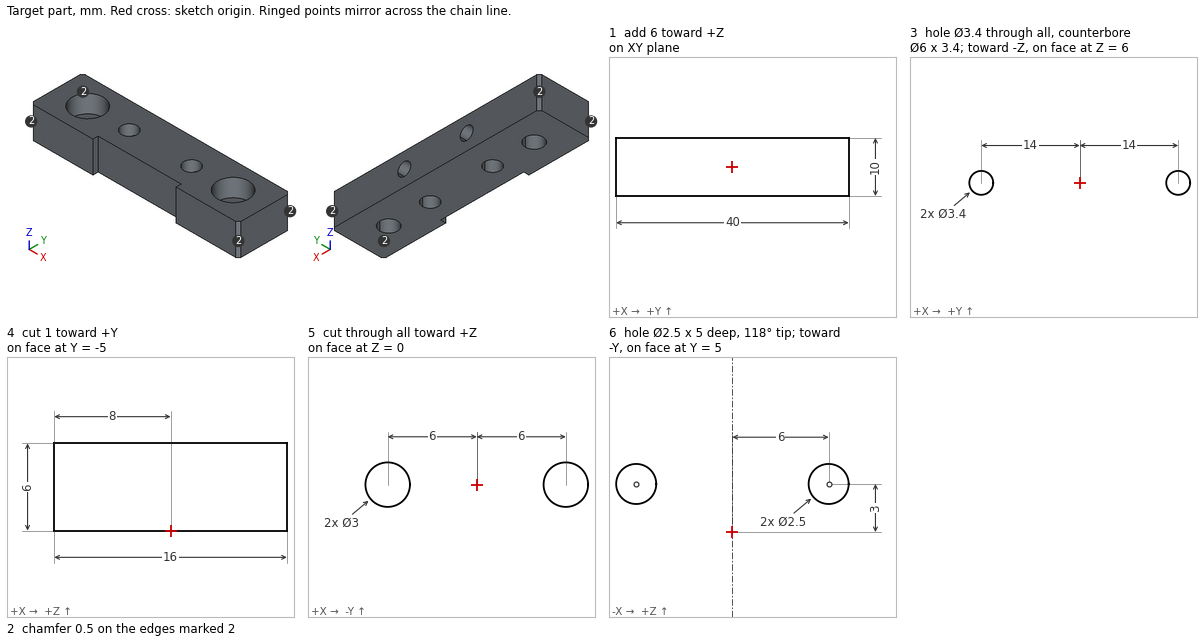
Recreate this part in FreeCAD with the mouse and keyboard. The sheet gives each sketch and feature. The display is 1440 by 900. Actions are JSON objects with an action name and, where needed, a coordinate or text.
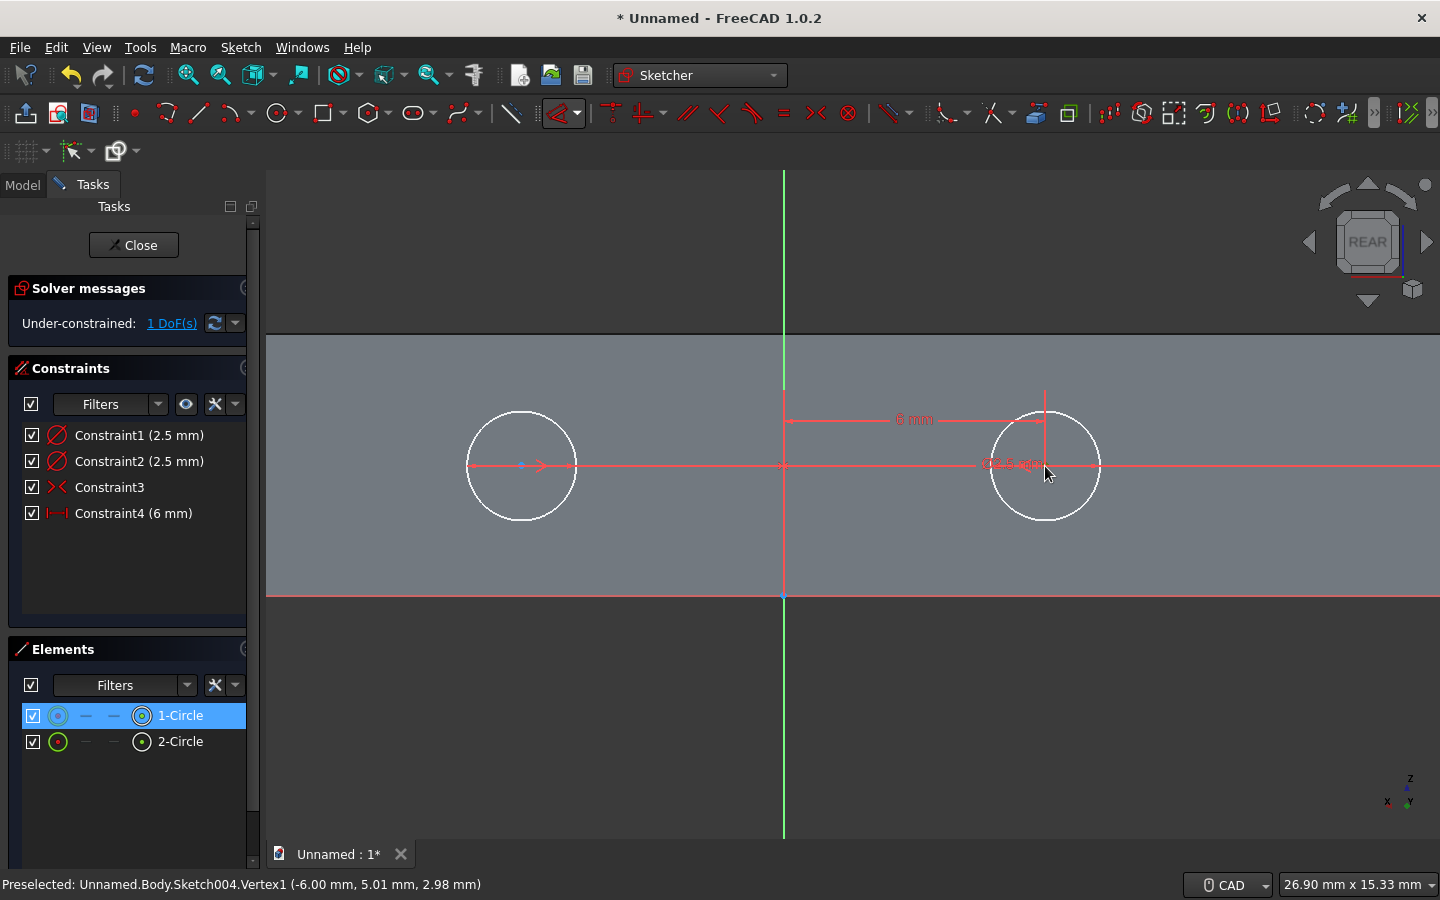
{"action": "left_click", "coordinate": [580, 114]}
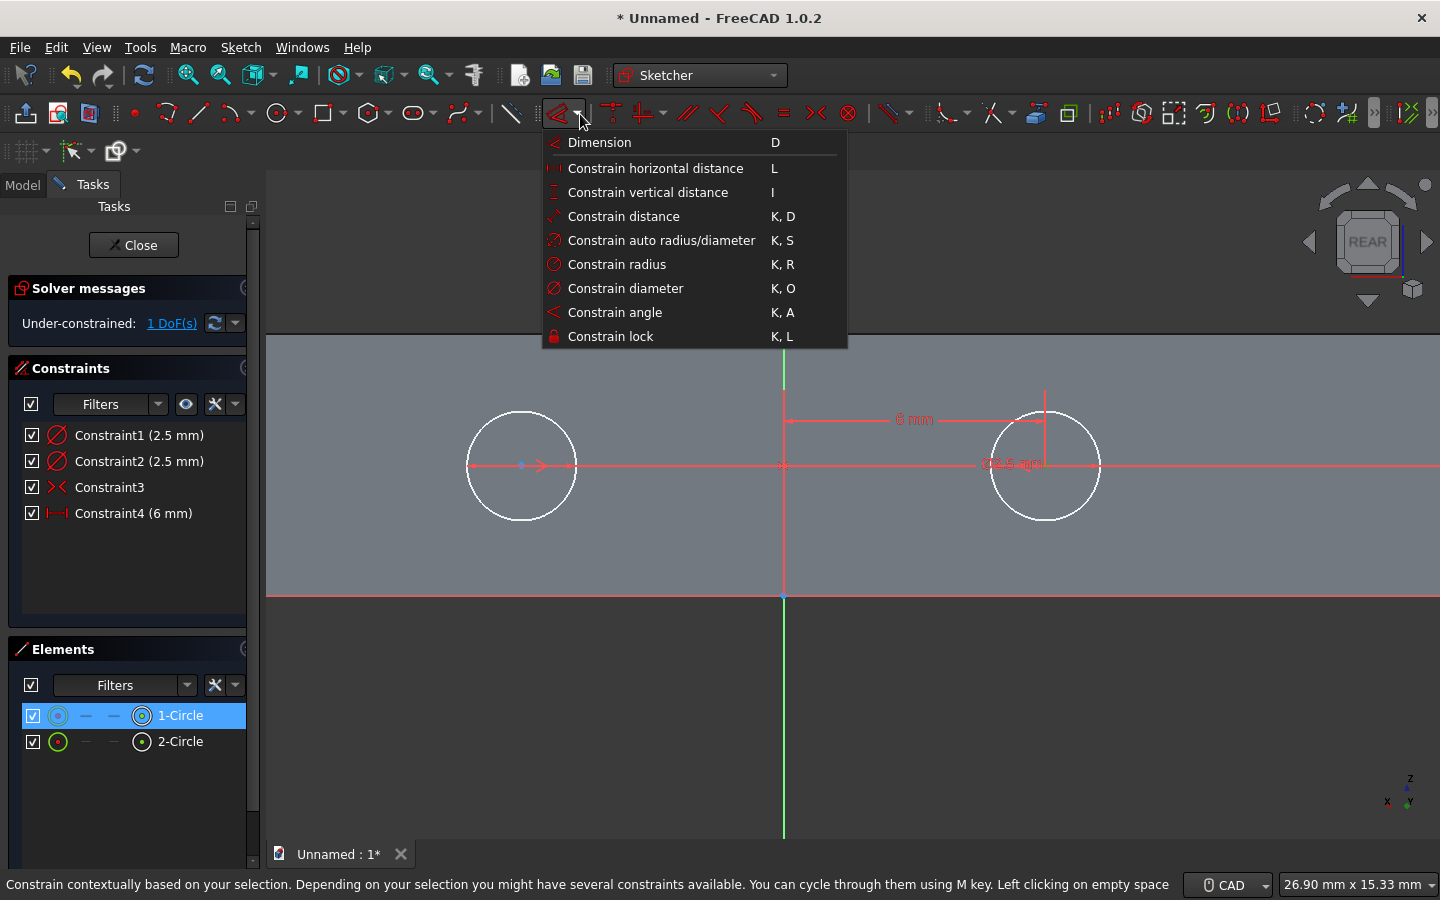
{"action": "left_click", "coordinate": [695, 192]}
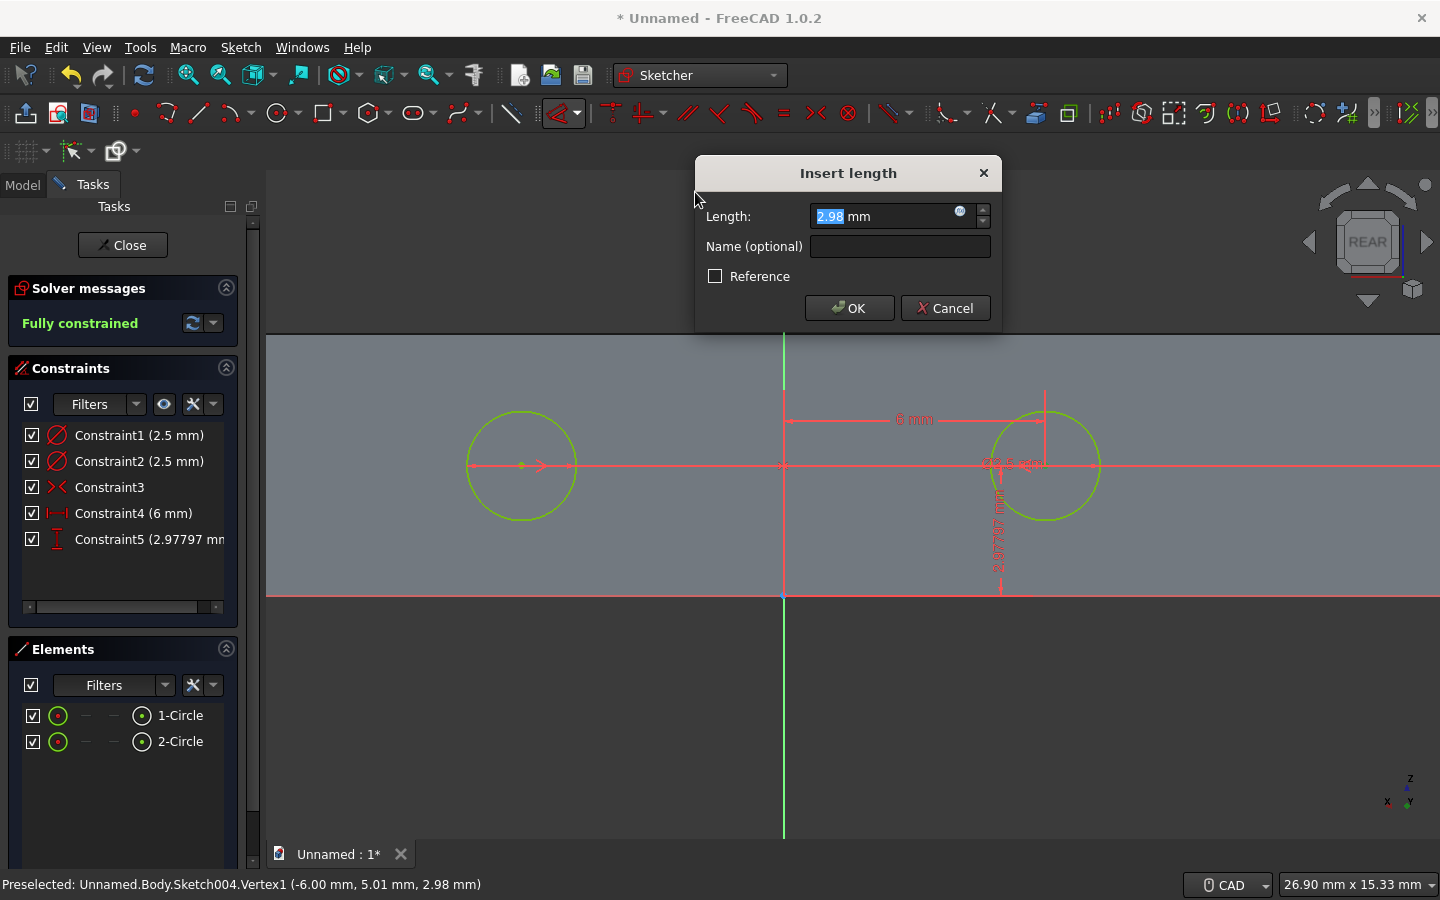
{"action": "type", "text": "3"}
{"action": "key", "text": "Return"}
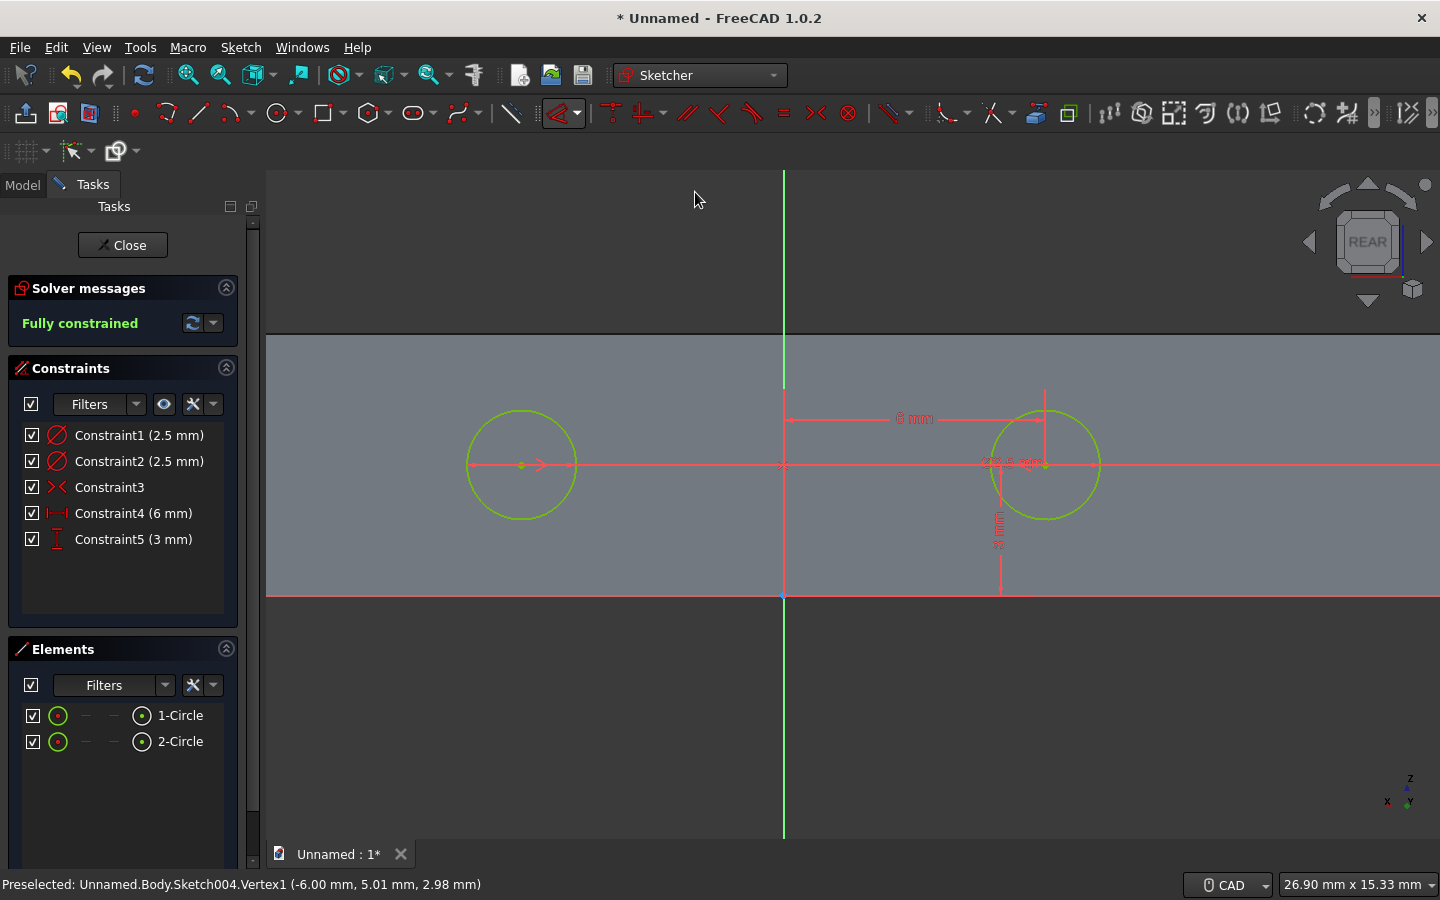
{"action": "left_click", "coordinate": [123, 245]}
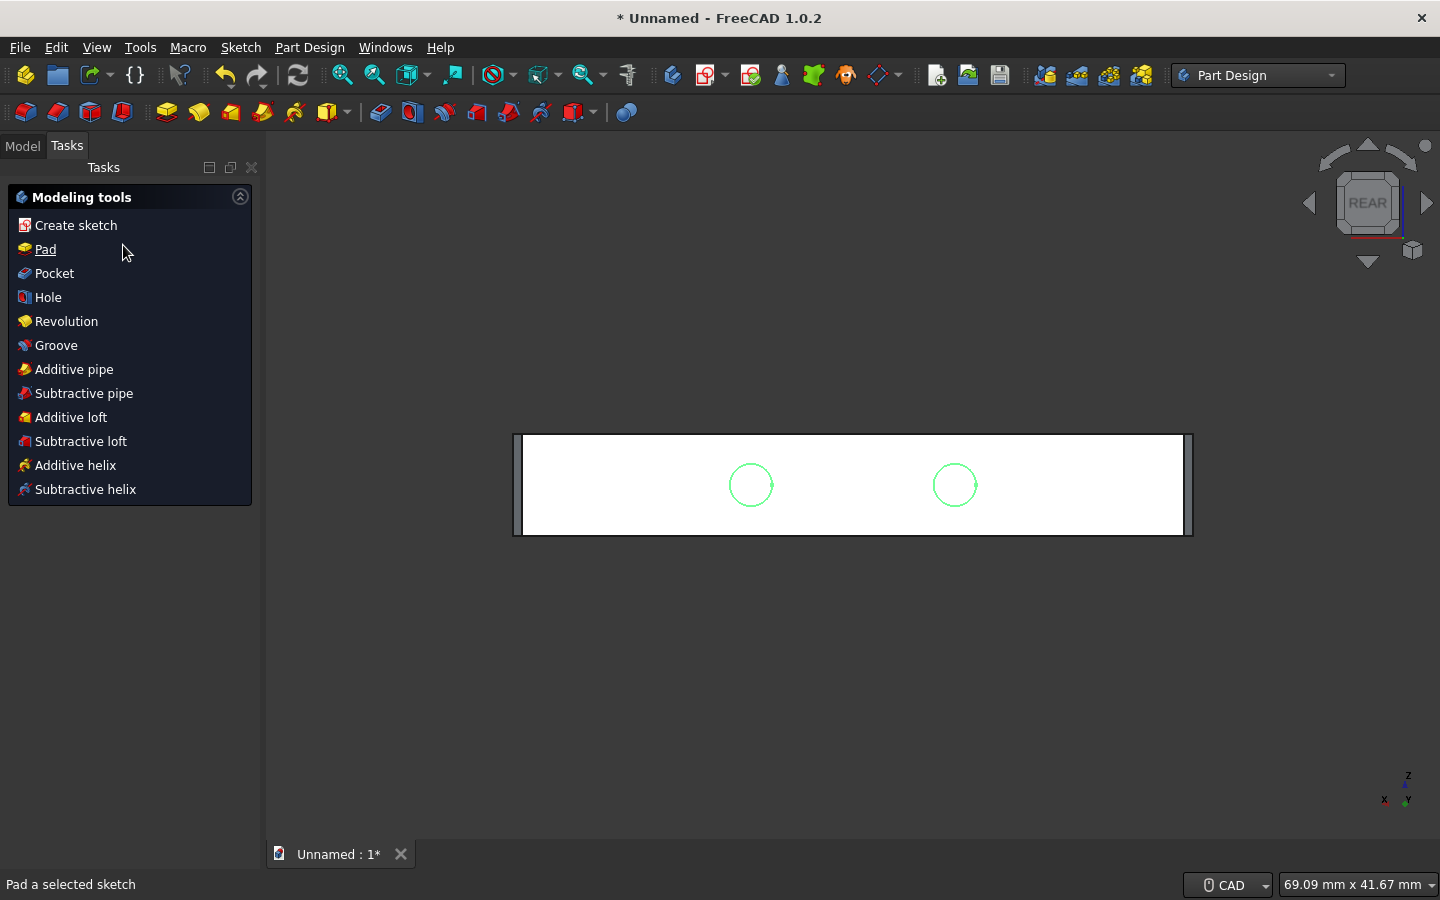
{"action": "left_click", "coordinate": [414, 112]}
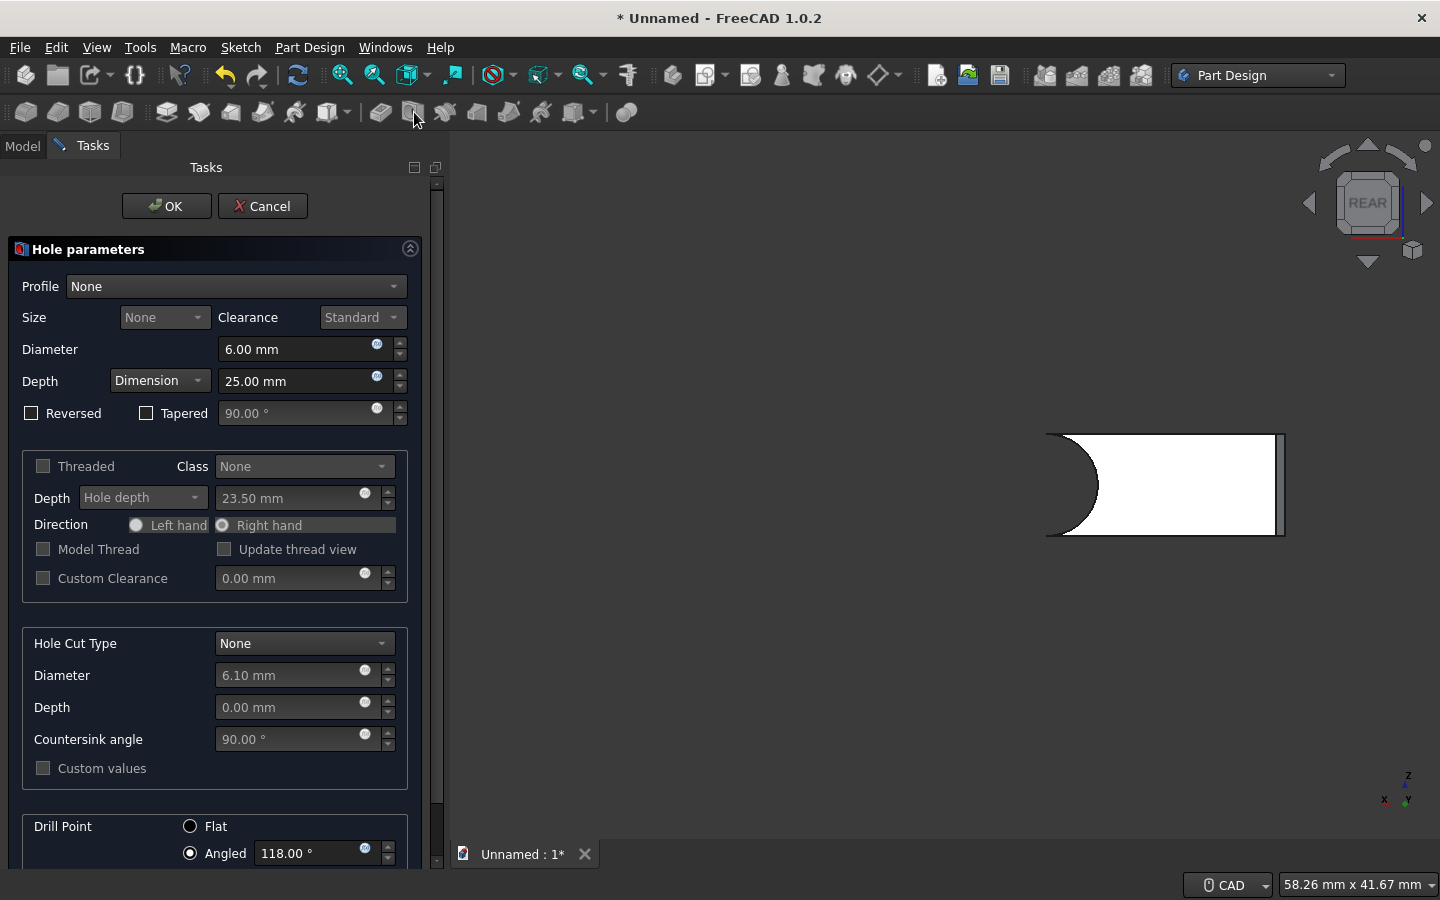
{"action": "triple_click", "coordinate": [305, 349]}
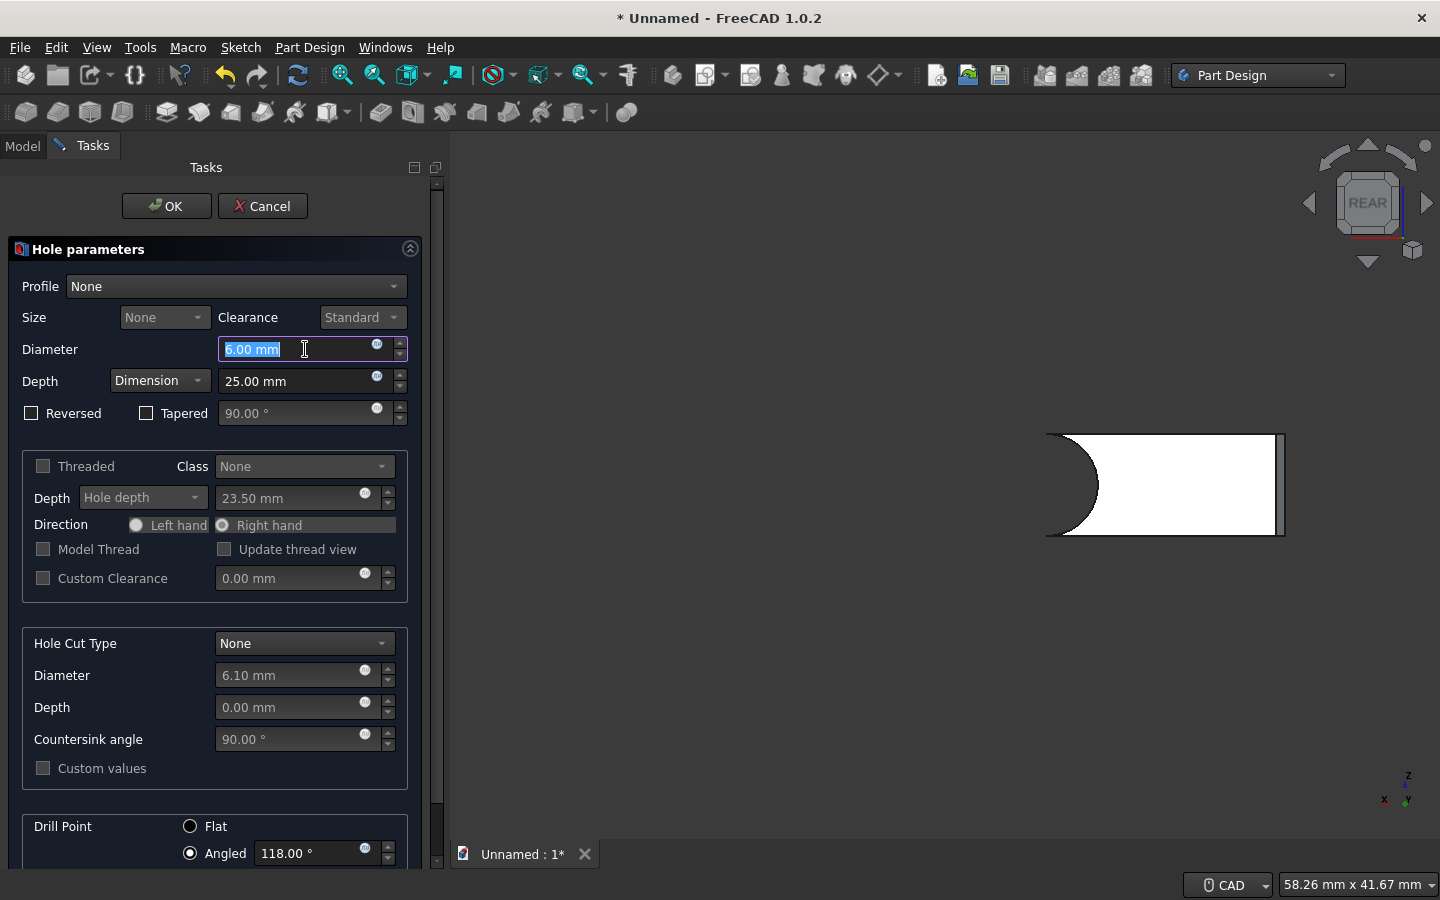
{"action": "type", "text": "2.5"}
{"action": "key", "text": "Tab"}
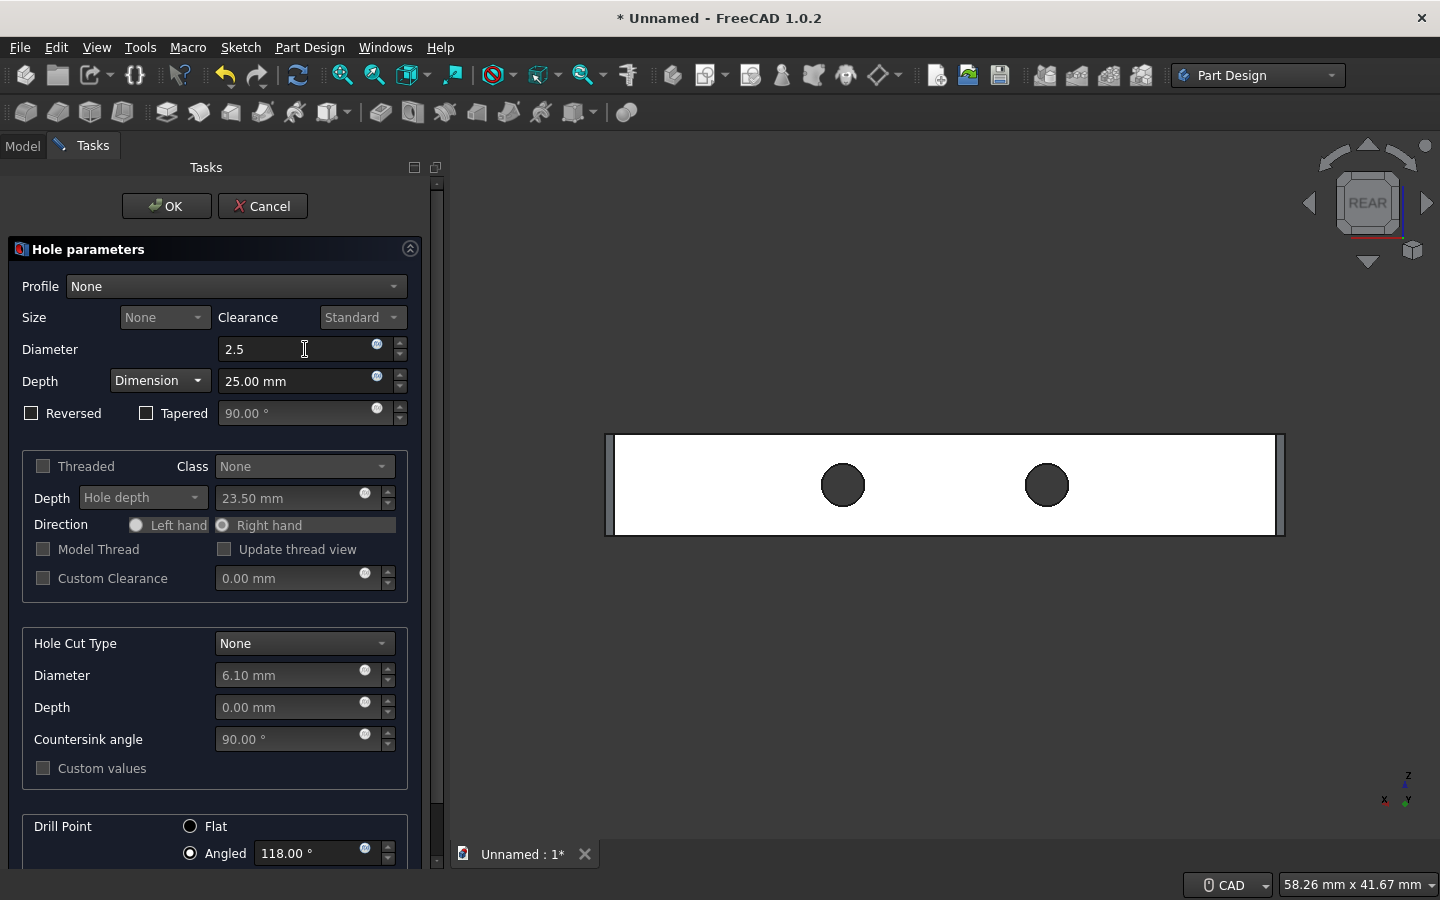
{"action": "triple_click", "coordinate": [305, 381]}